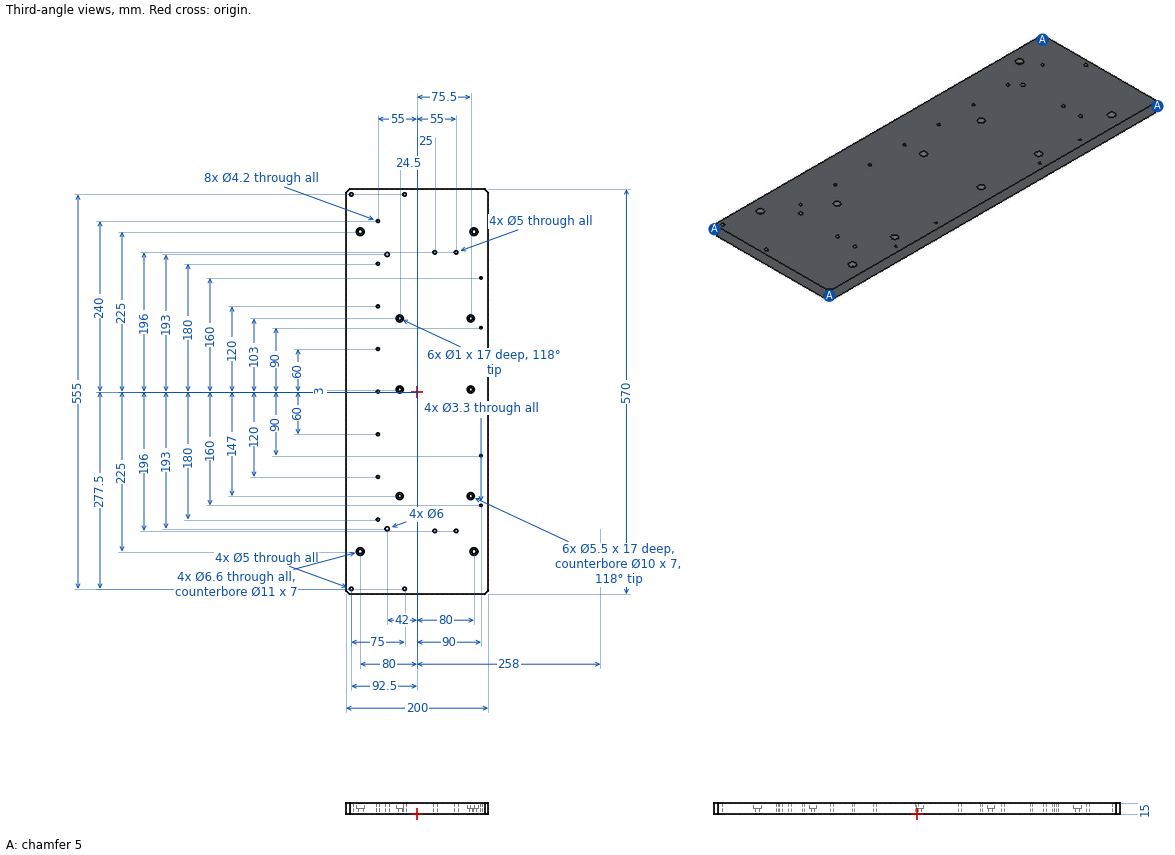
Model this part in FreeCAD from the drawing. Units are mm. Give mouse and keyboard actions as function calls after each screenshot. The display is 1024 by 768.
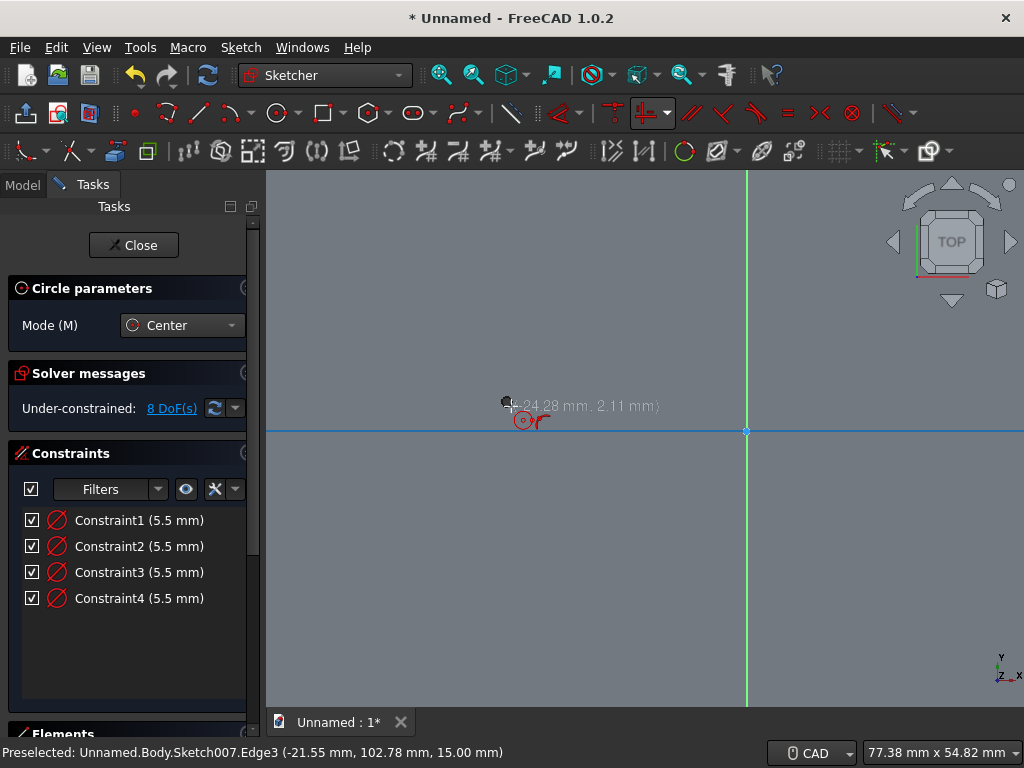
click(507, 402)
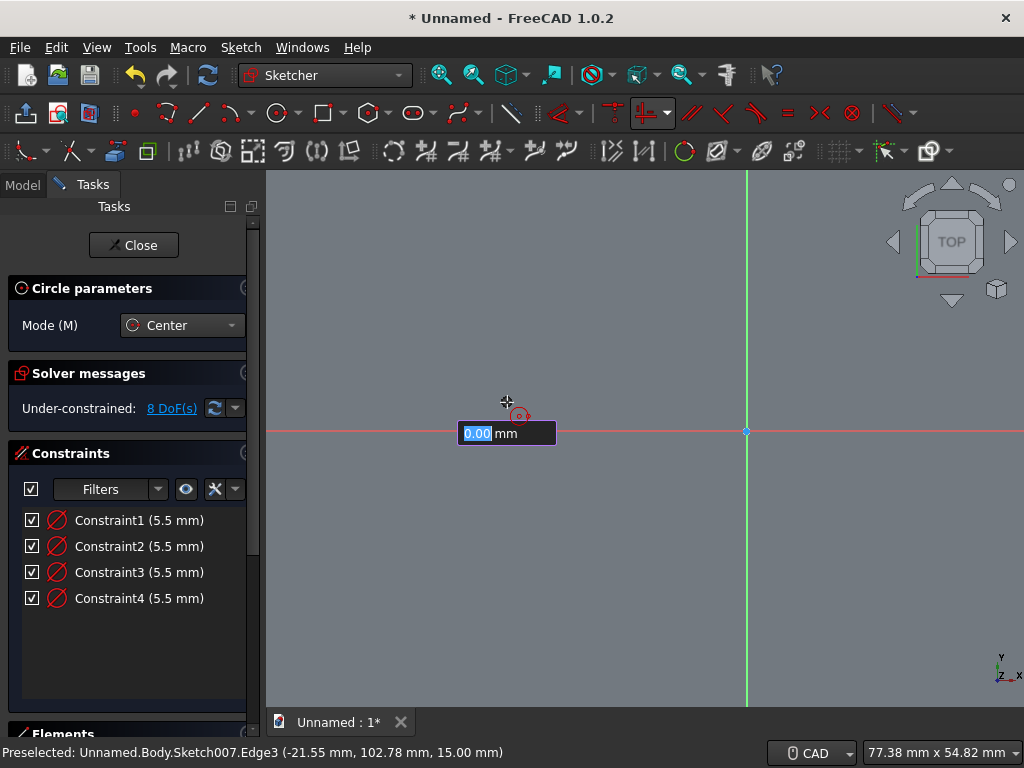
scroll(511, 406, down, 10)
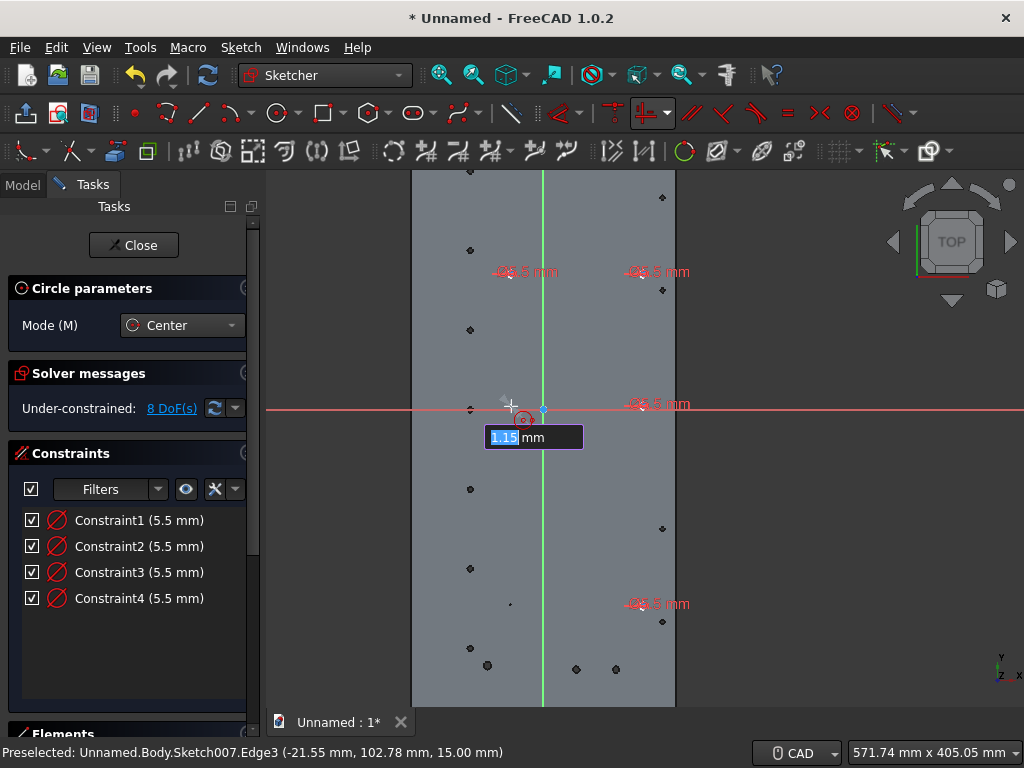
scroll(513, 403, up, 5)
move(513, 403)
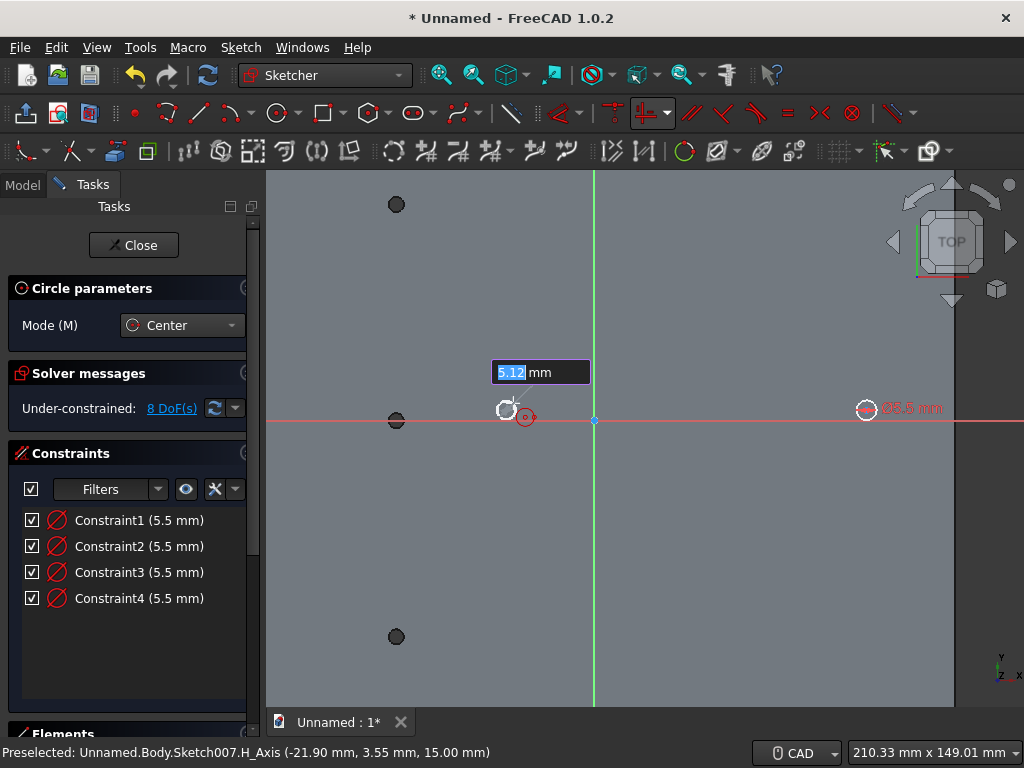
text(5.5)
key(Return)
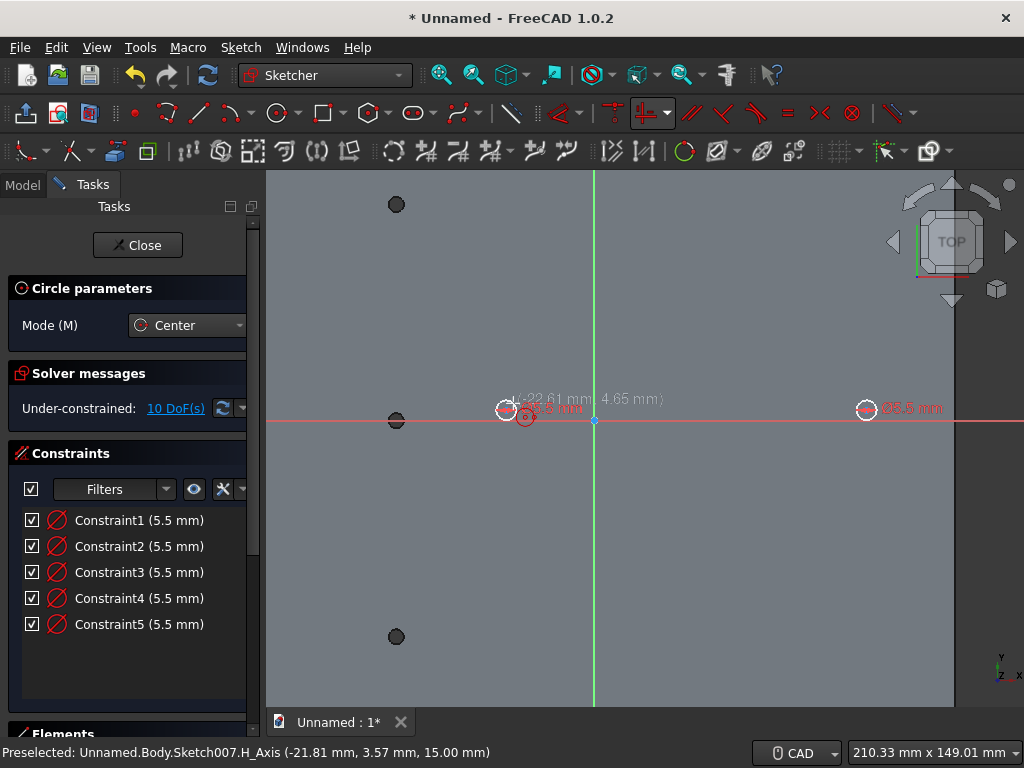
scroll(513, 403, down, 5)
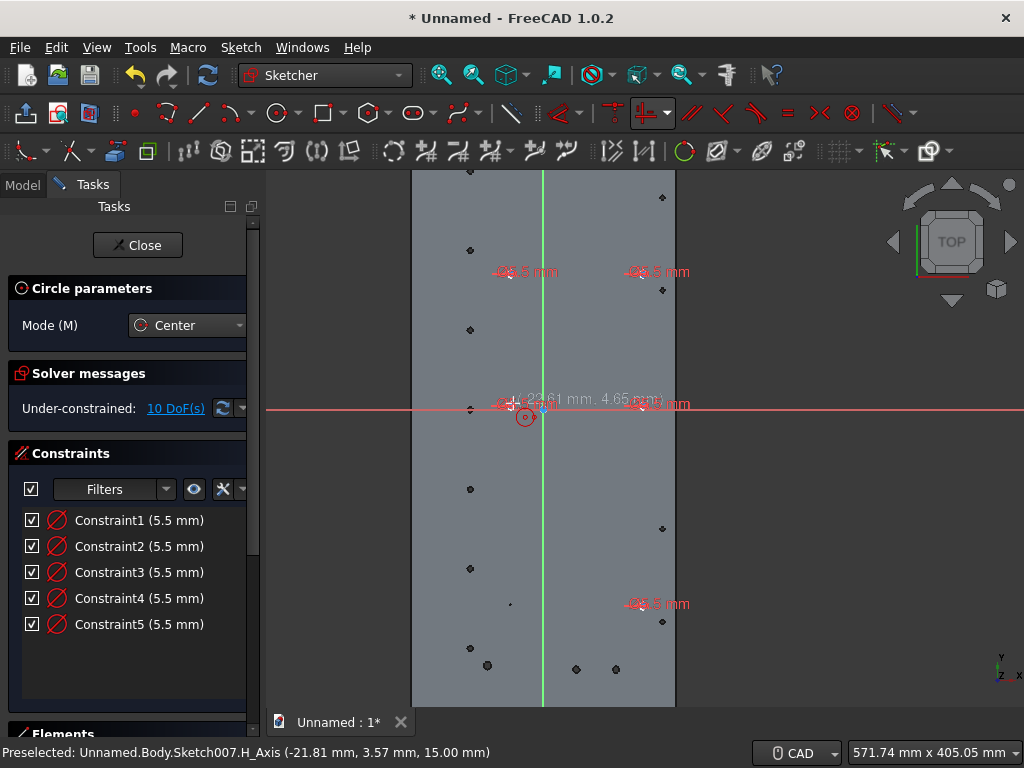
scroll(511, 605, up, 10)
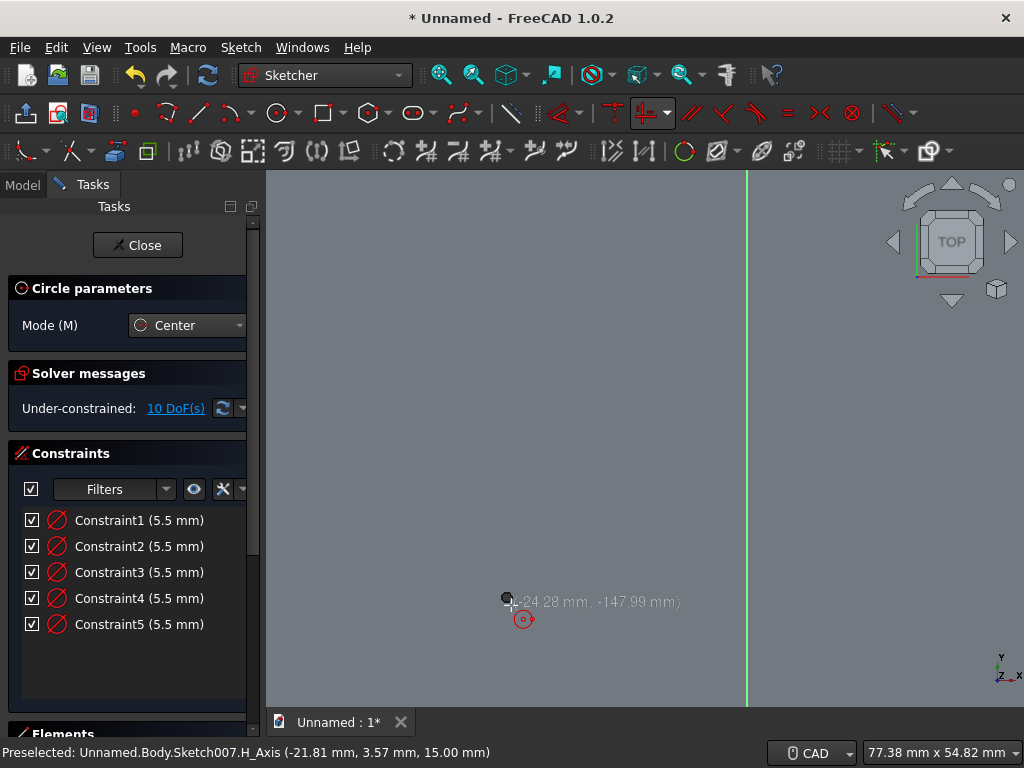
scroll(511, 605, down, 10)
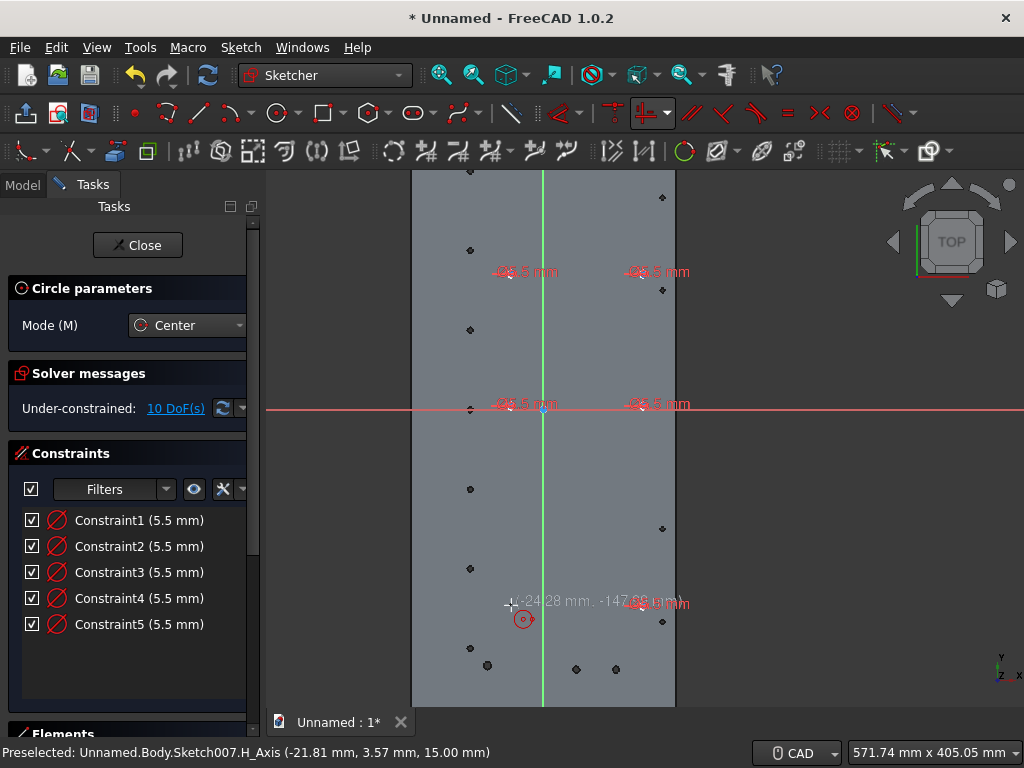
click(511, 605)
move(513, 602)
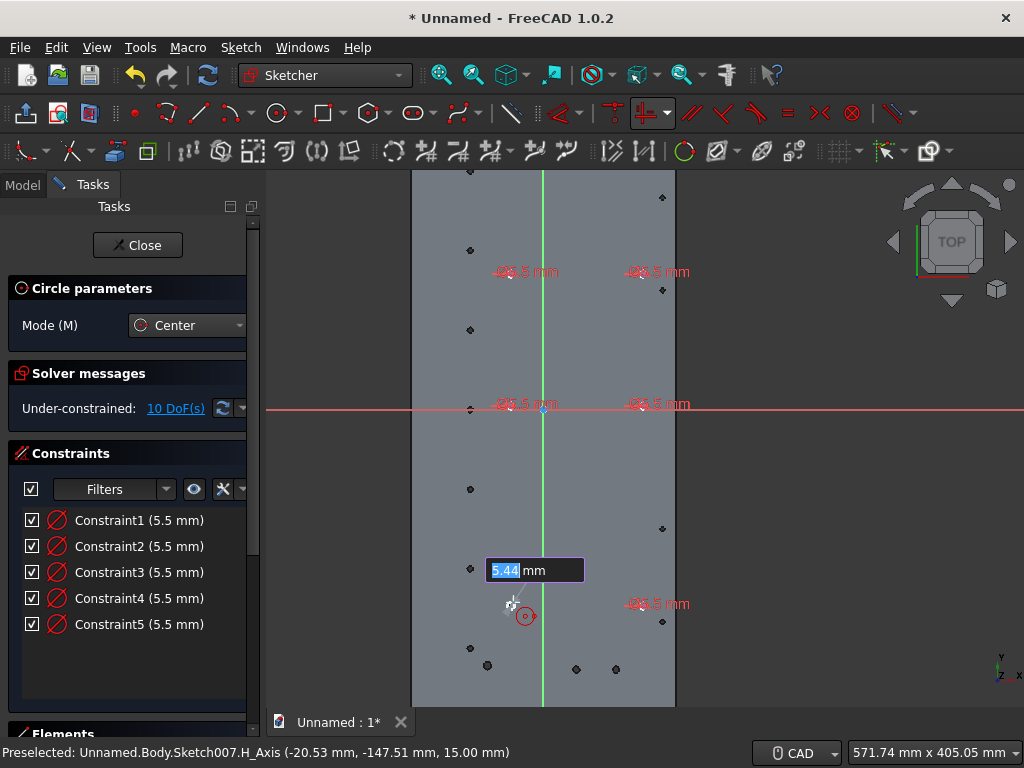
text(5.5)
key(Return)
key(Escape)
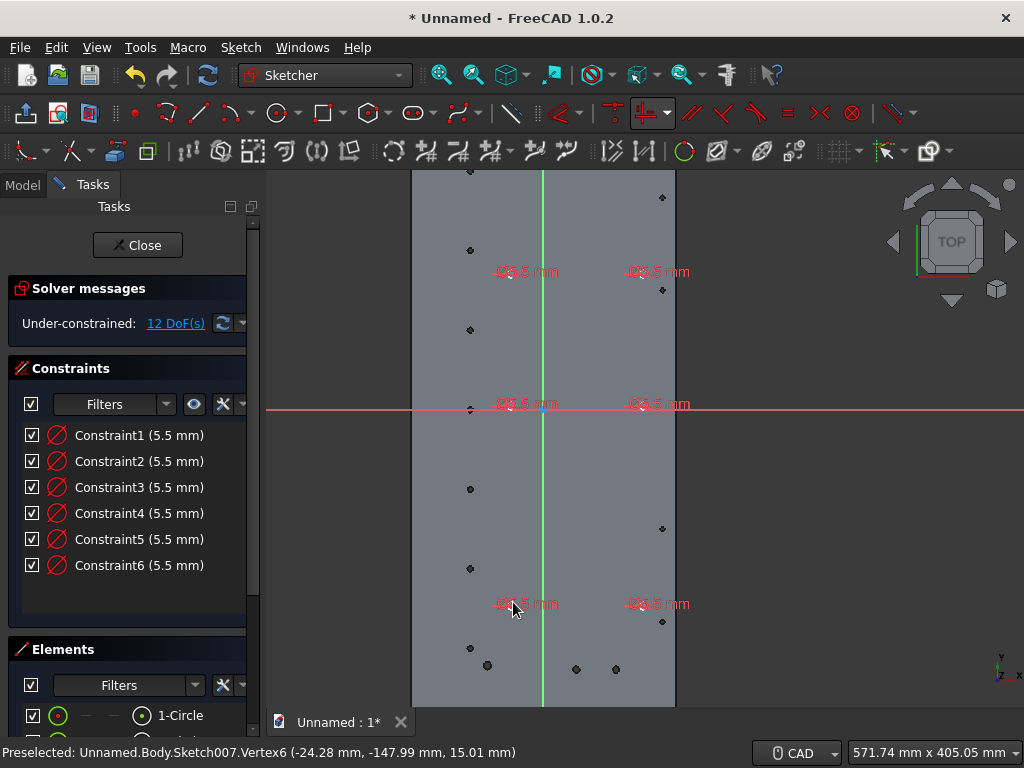
click(643, 606)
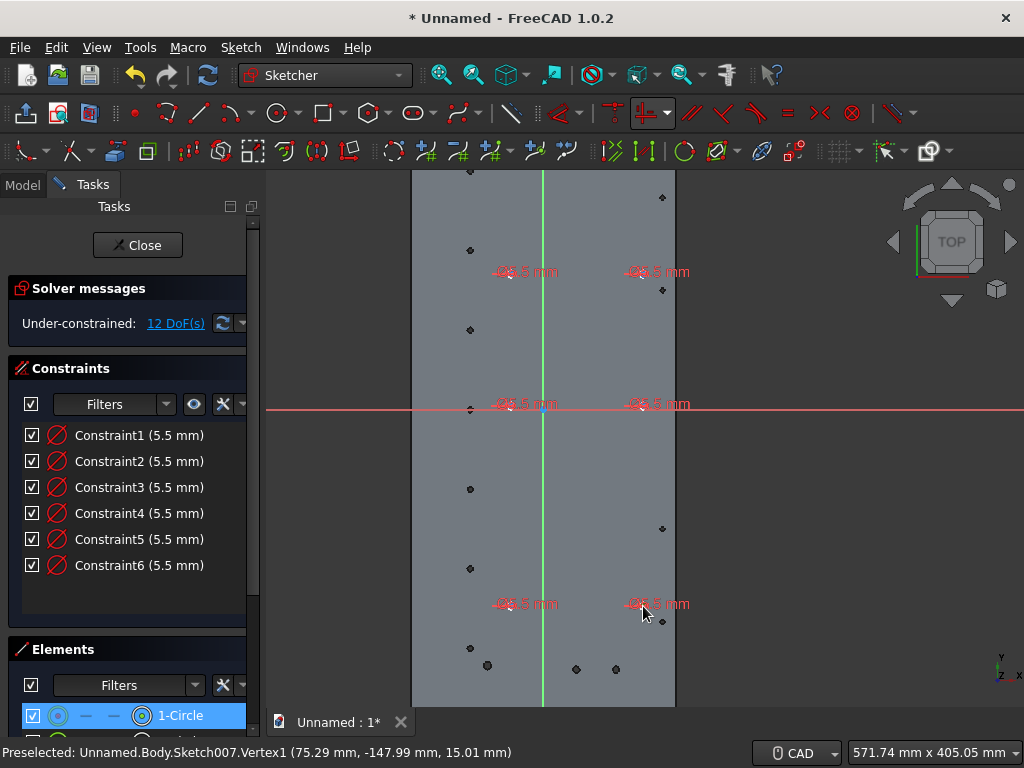
click(643, 274)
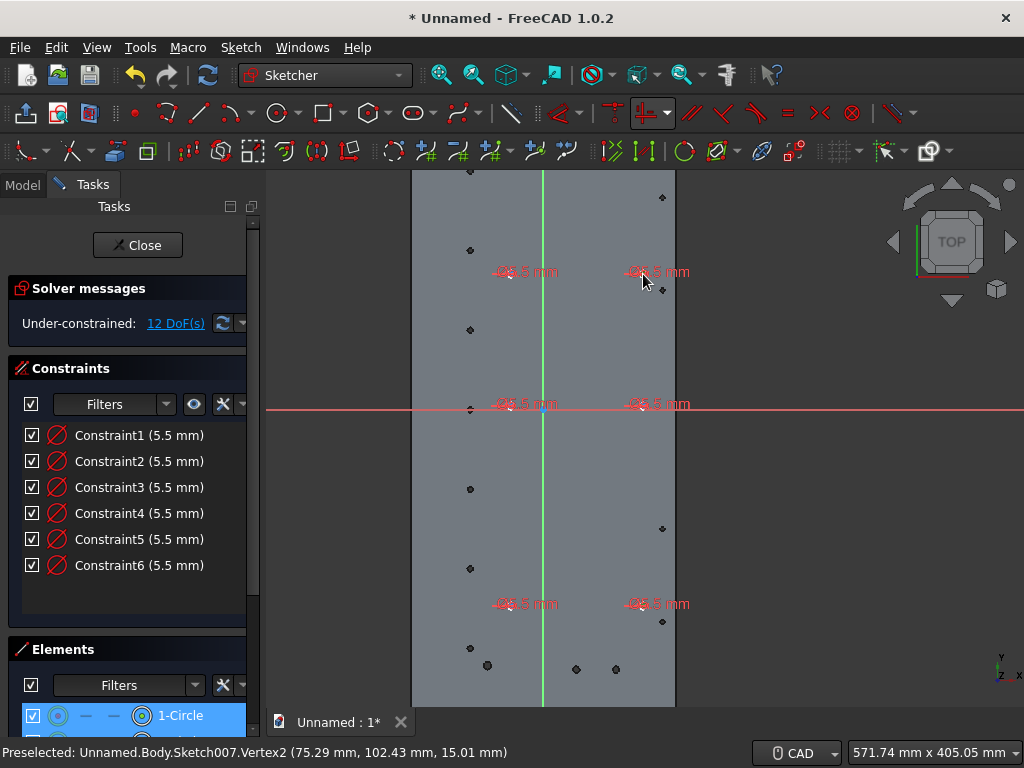
key(v)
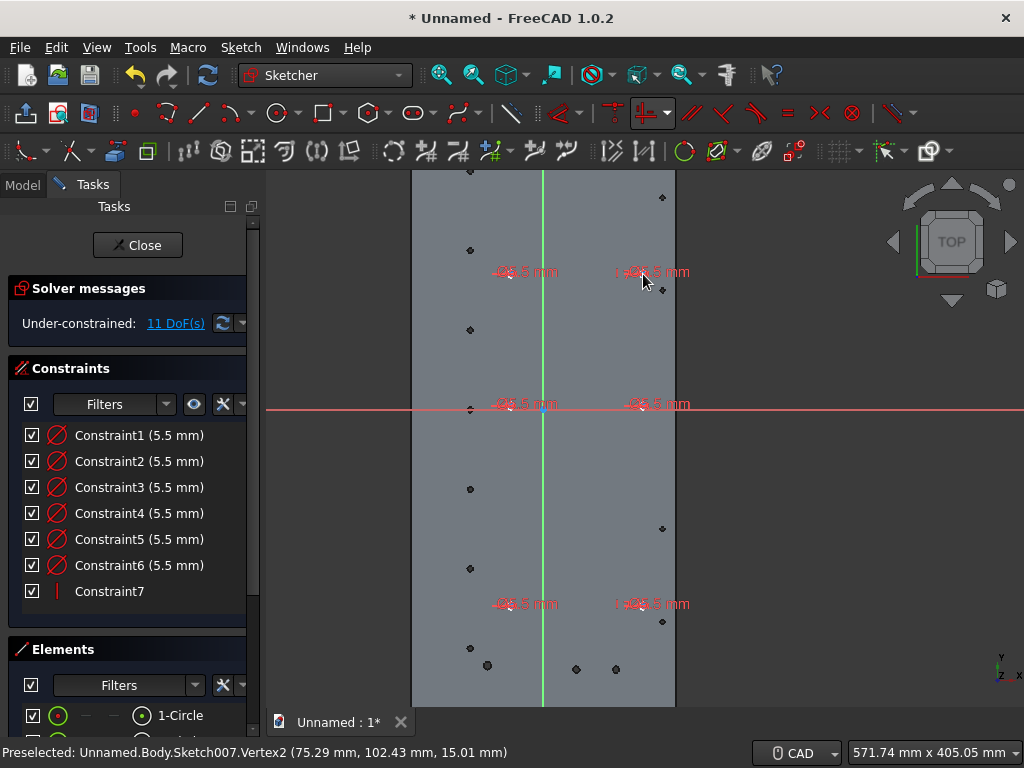
click(643, 274)